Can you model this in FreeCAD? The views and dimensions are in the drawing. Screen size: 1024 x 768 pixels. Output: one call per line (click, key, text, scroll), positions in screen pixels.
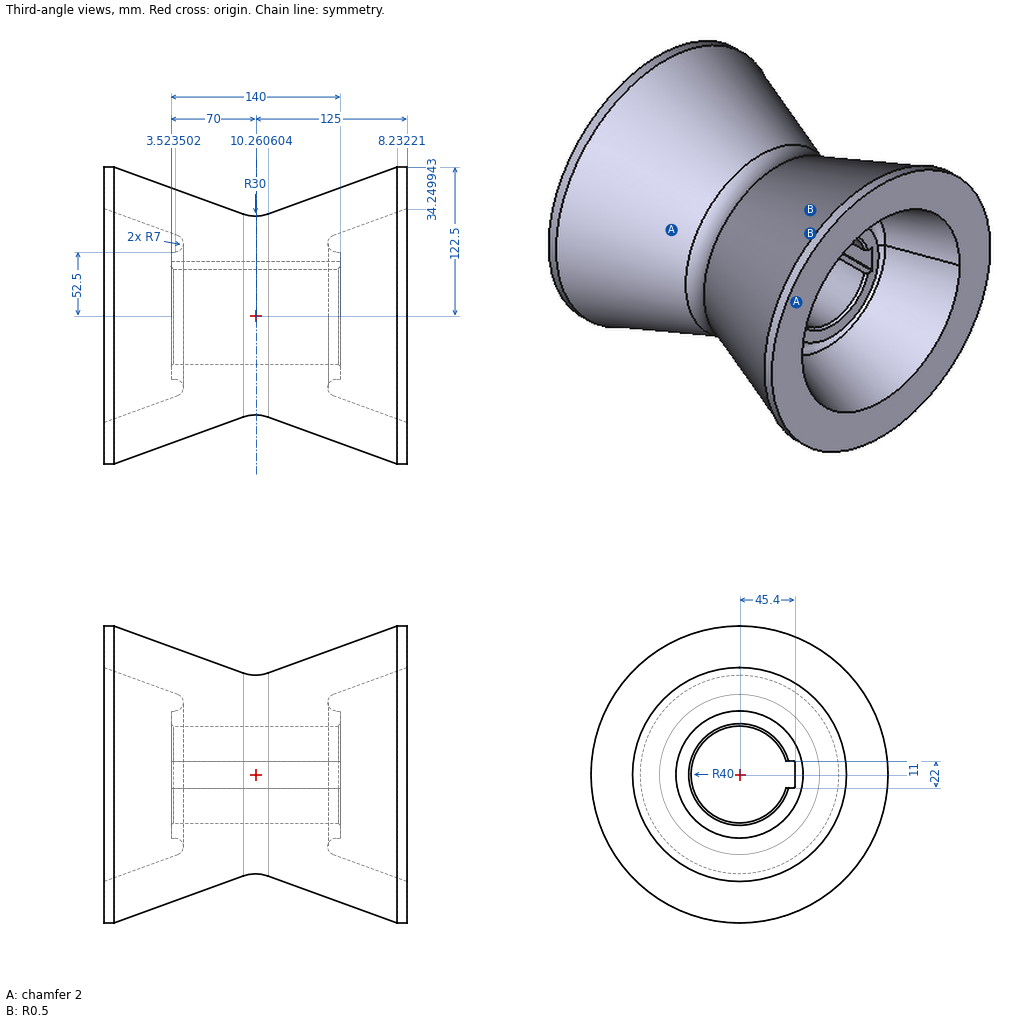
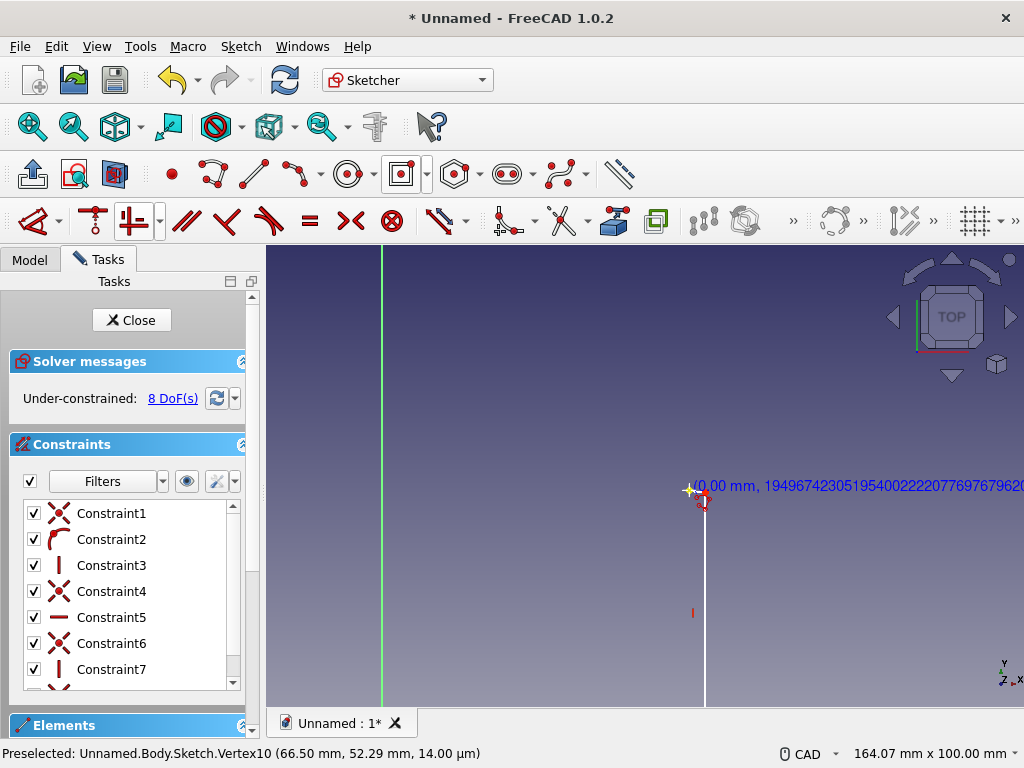
click(678, 427)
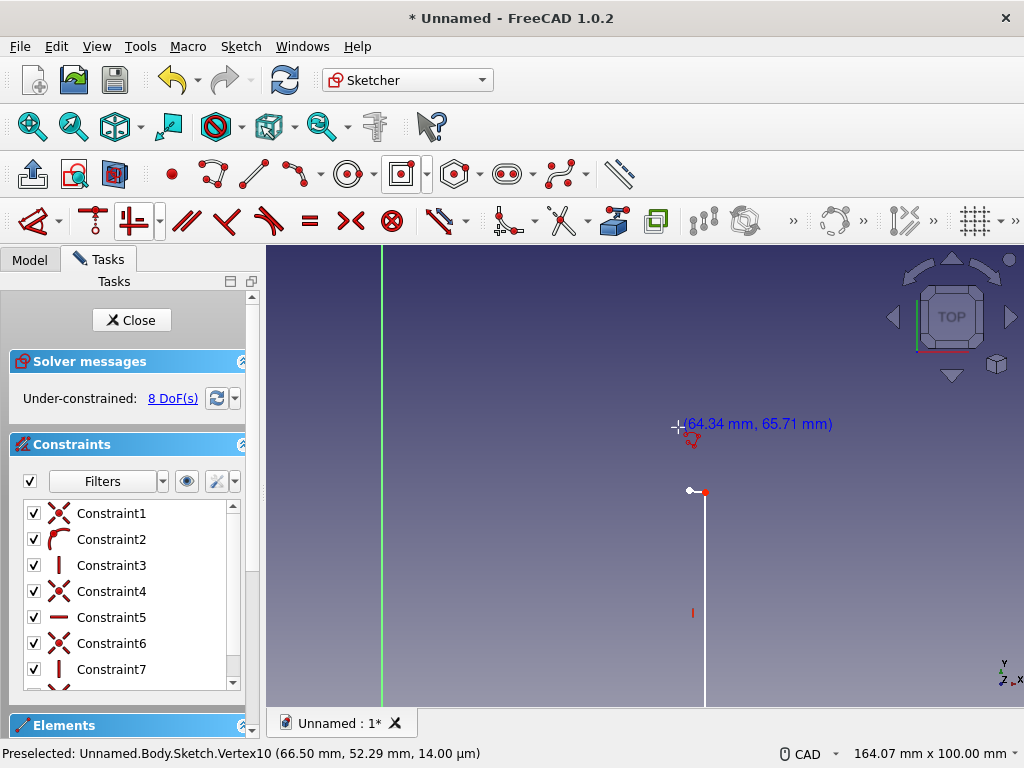
scroll(690, 491, down, 5)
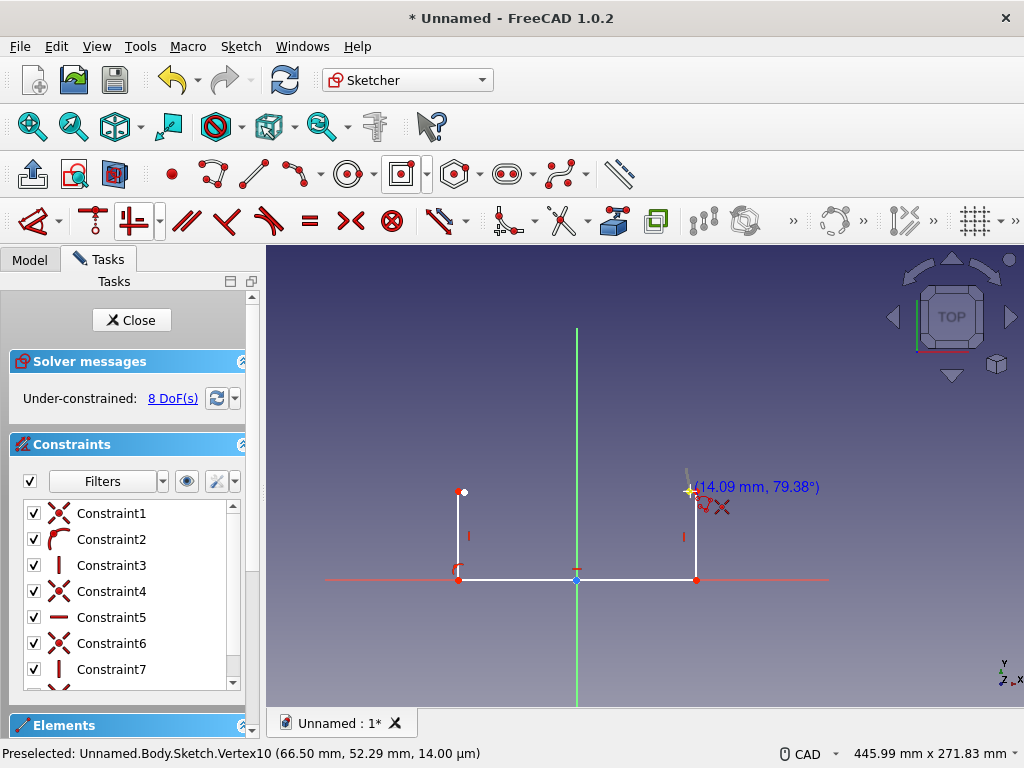
click(789, 430)
click(789, 372)
click(775, 372)
click(594, 438)
right_click(594, 438)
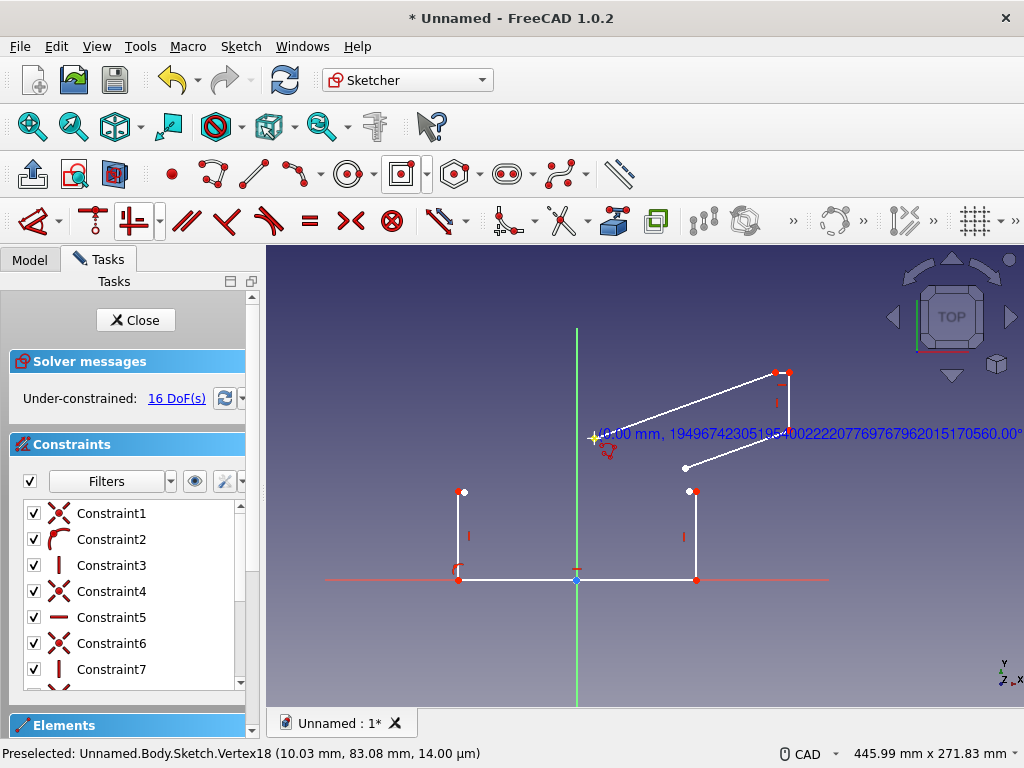
click(560, 438)
click(378, 372)
click(365, 372)
click(365, 430)
click(468, 468)
right_click(468, 468)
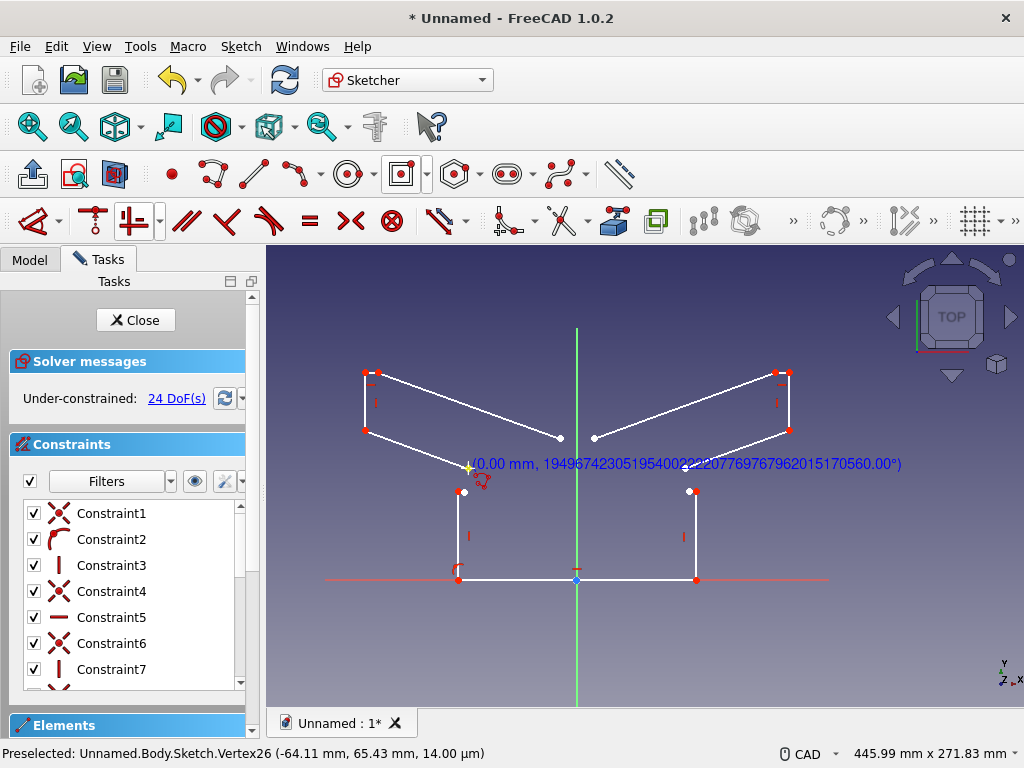
click(294, 174)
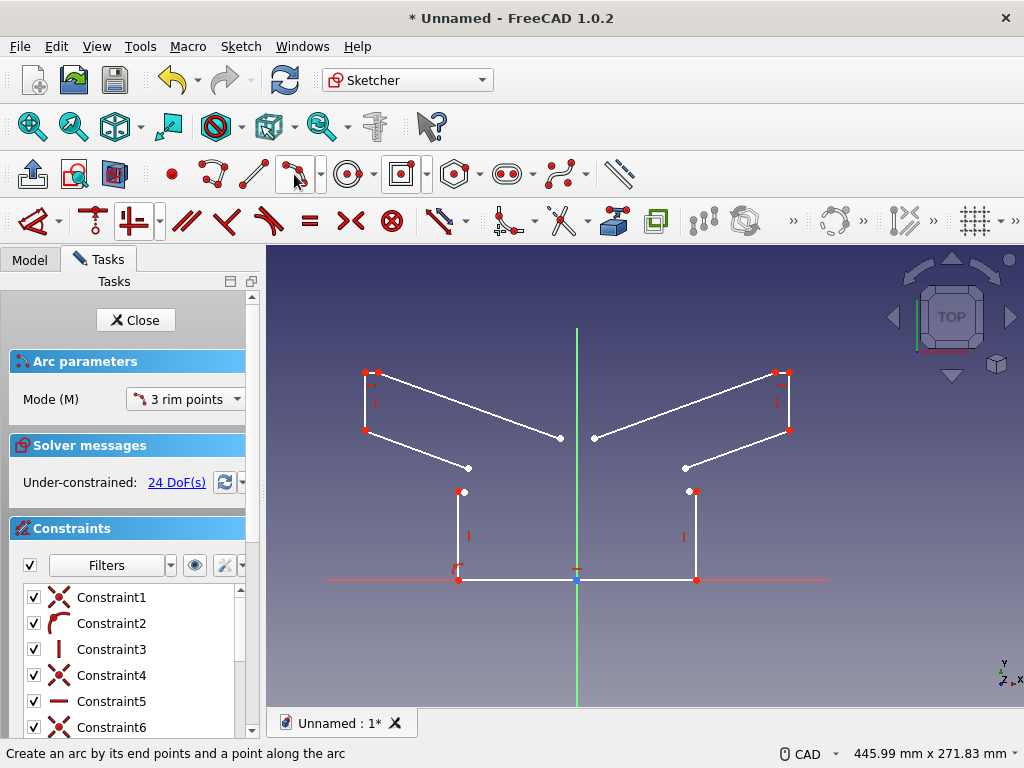
scroll(690, 491, up, 9)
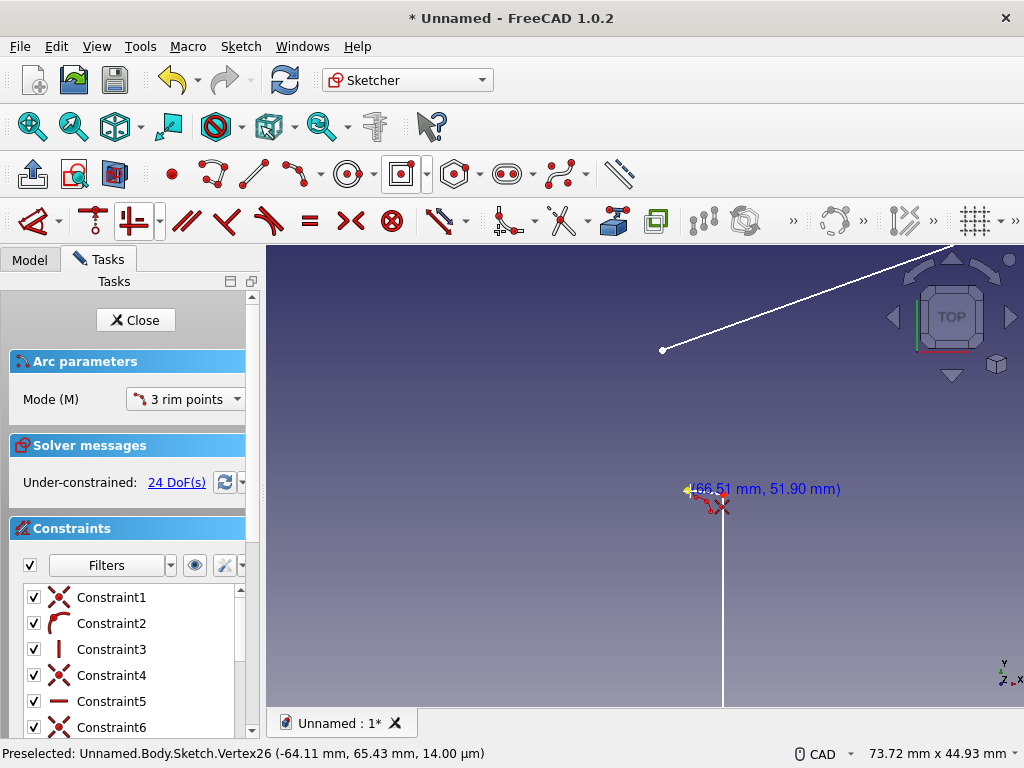
click(687, 490)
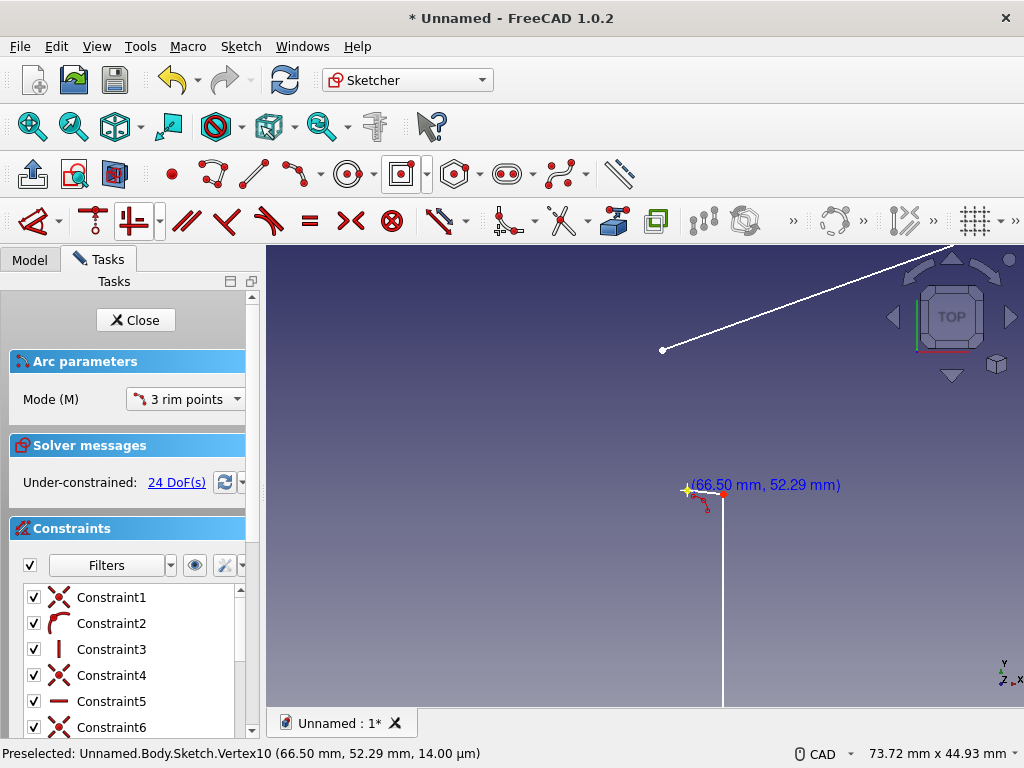
scroll(690, 491, down, 9)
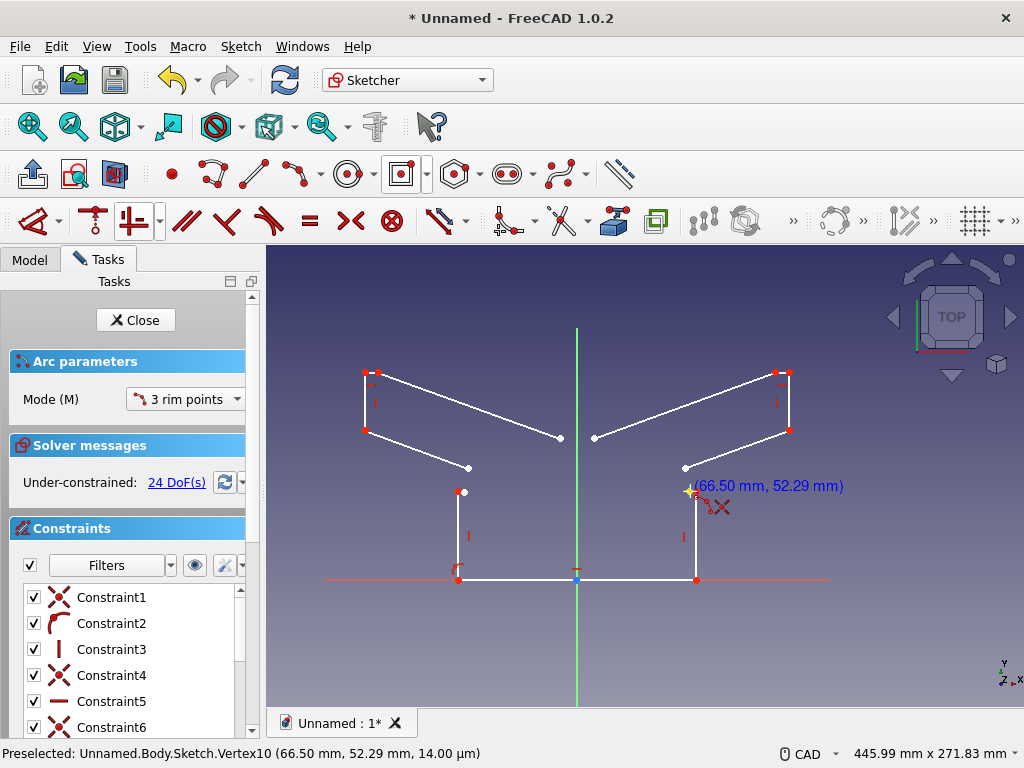
click(686, 468)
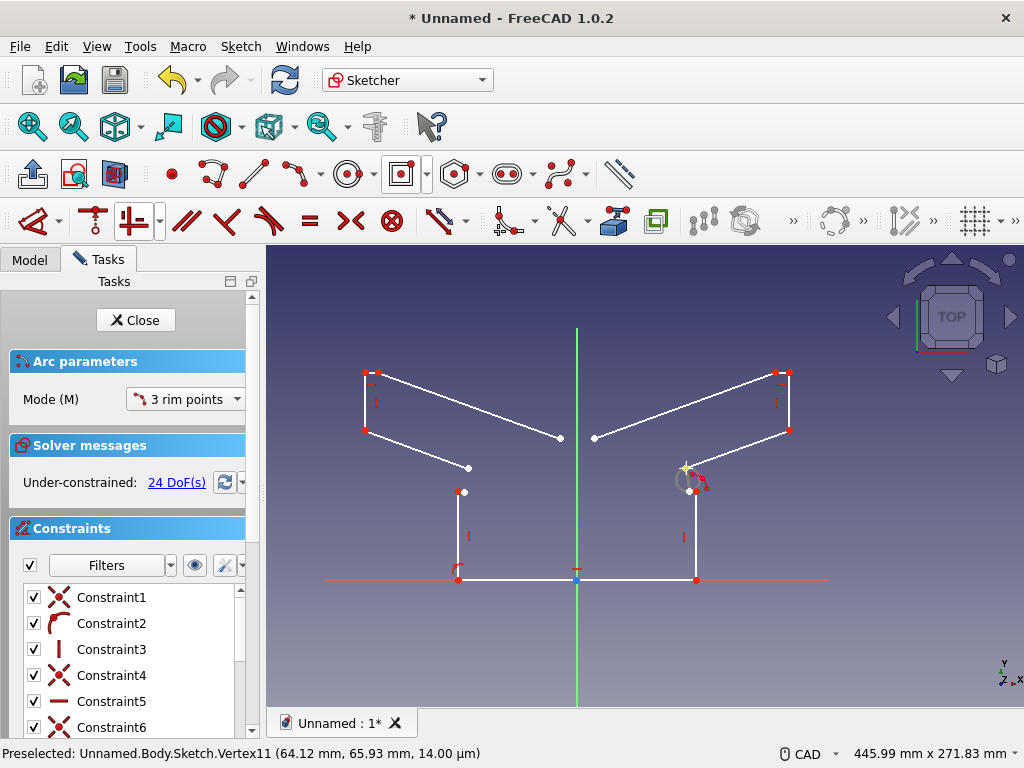
scroll(678, 481, up, 3)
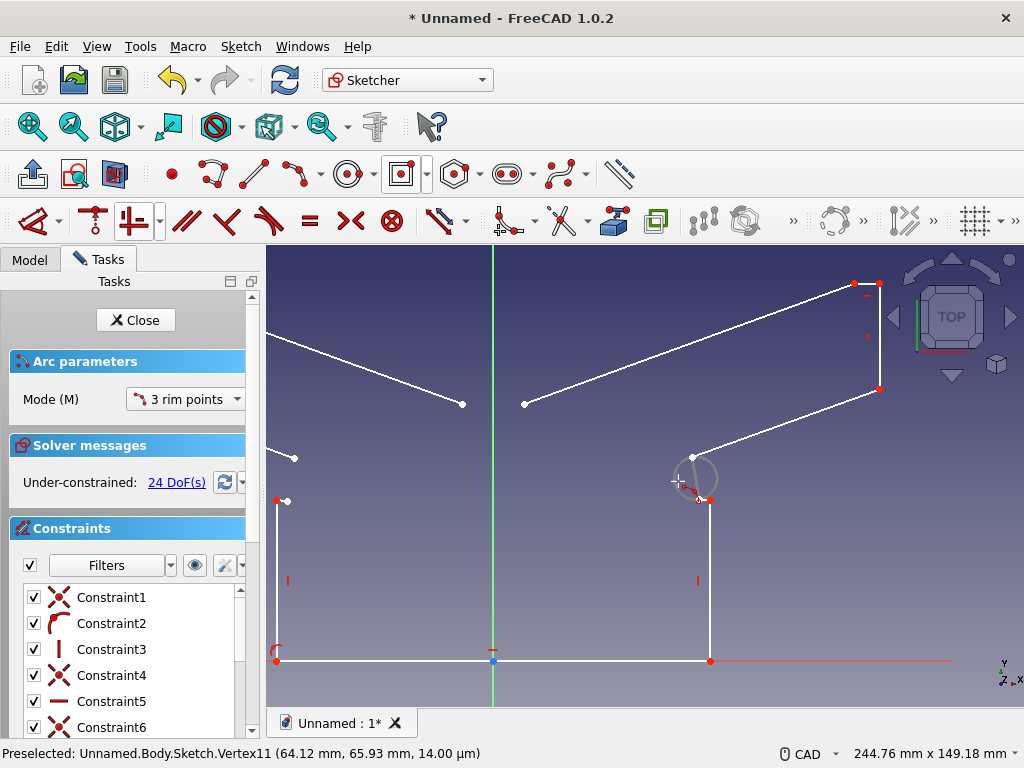
click(678, 481)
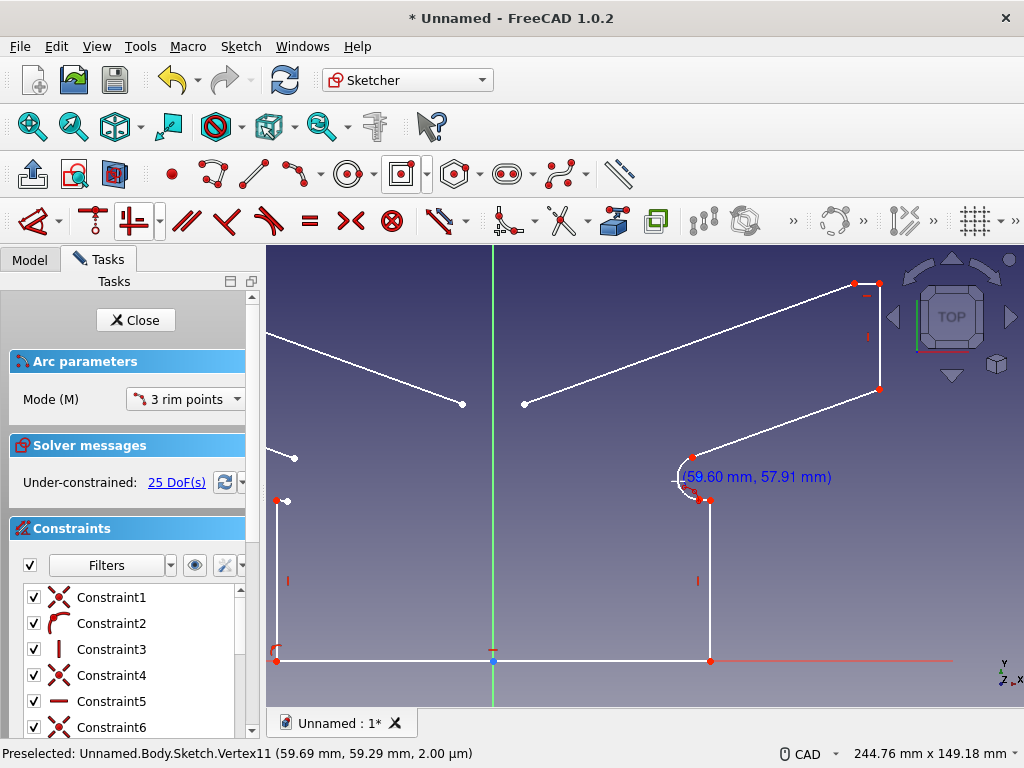
click(524, 404)
click(463, 404)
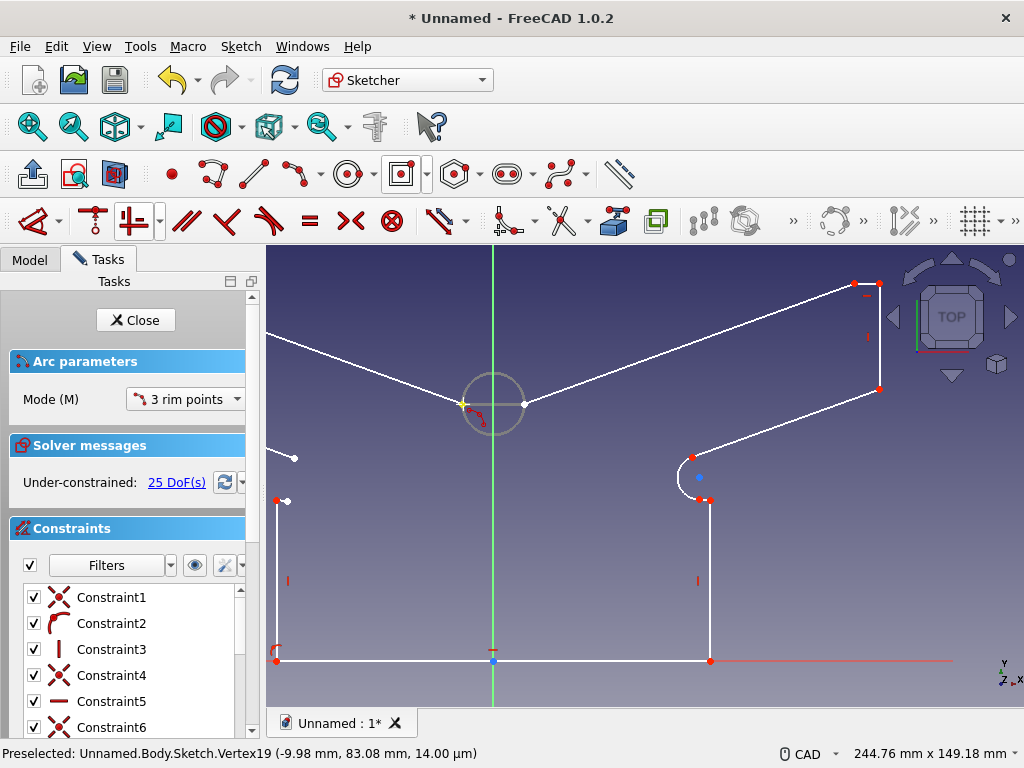
scroll(487, 407, up, 6)